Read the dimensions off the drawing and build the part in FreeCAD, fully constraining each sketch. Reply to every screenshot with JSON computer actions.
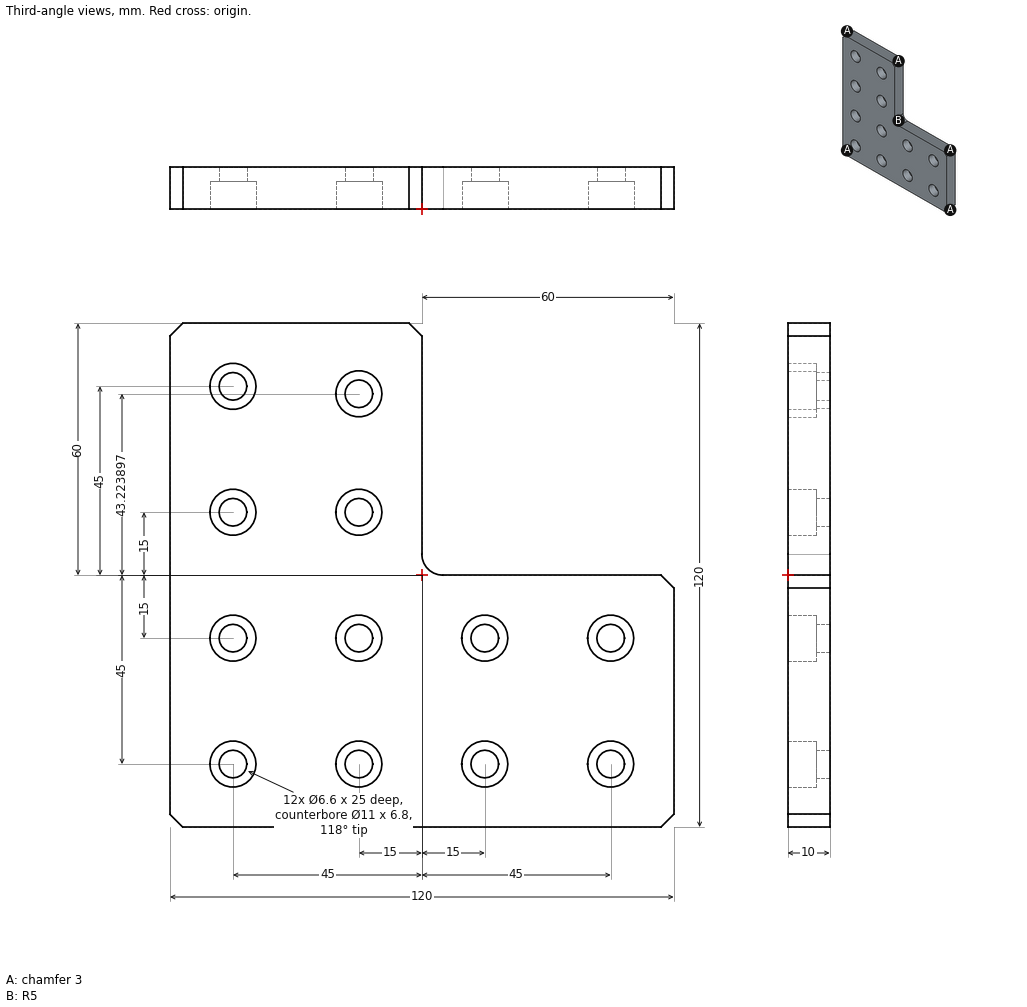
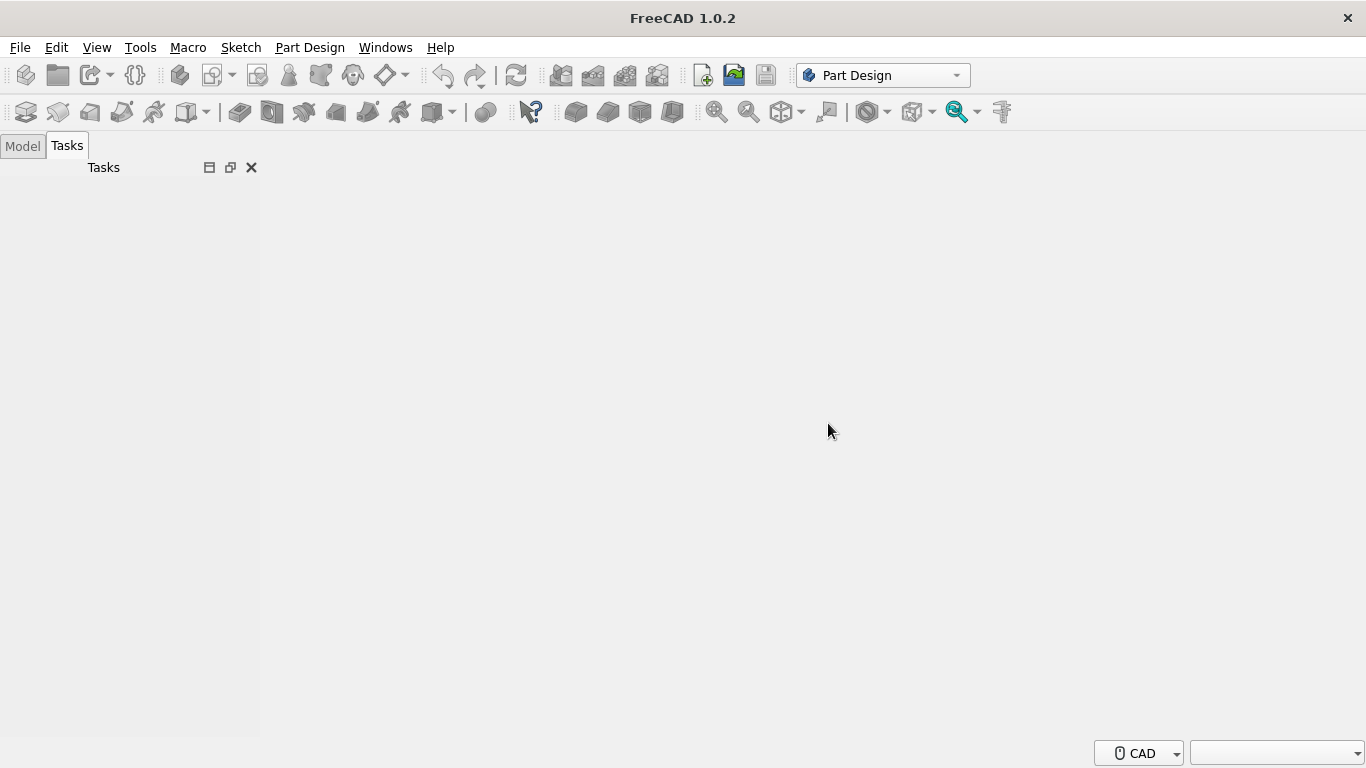
{"action": "left_click", "coordinate": [702, 76]}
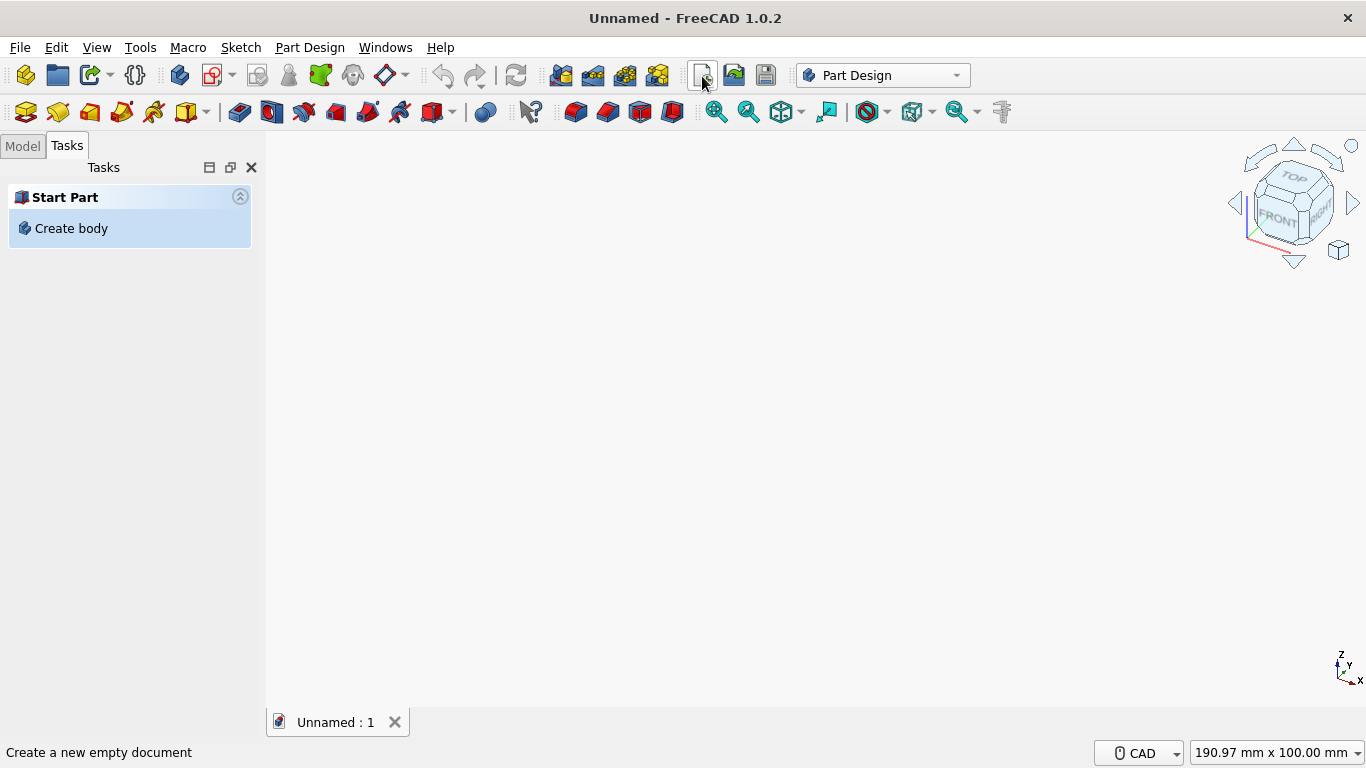
{"action": "left_click", "coordinate": [212, 76]}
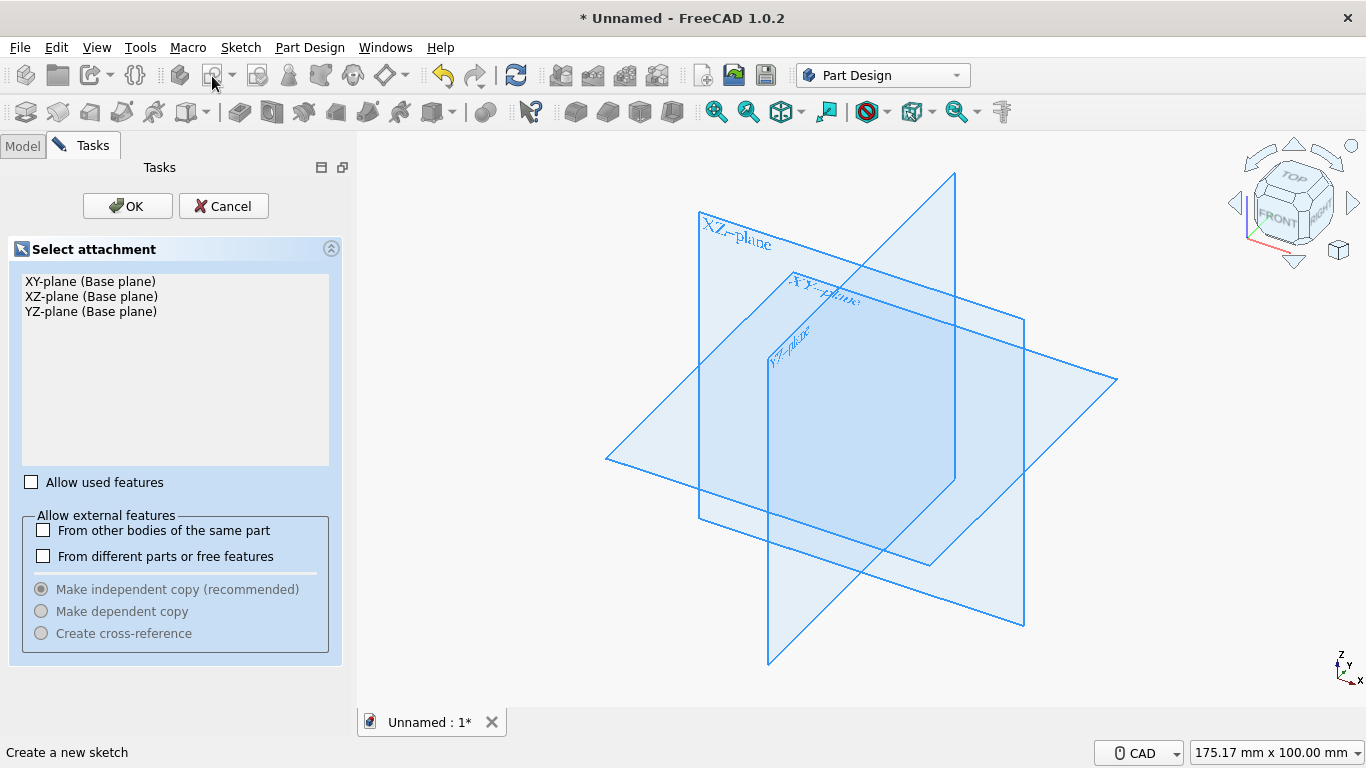
{"action": "left_click", "coordinate": [82, 296]}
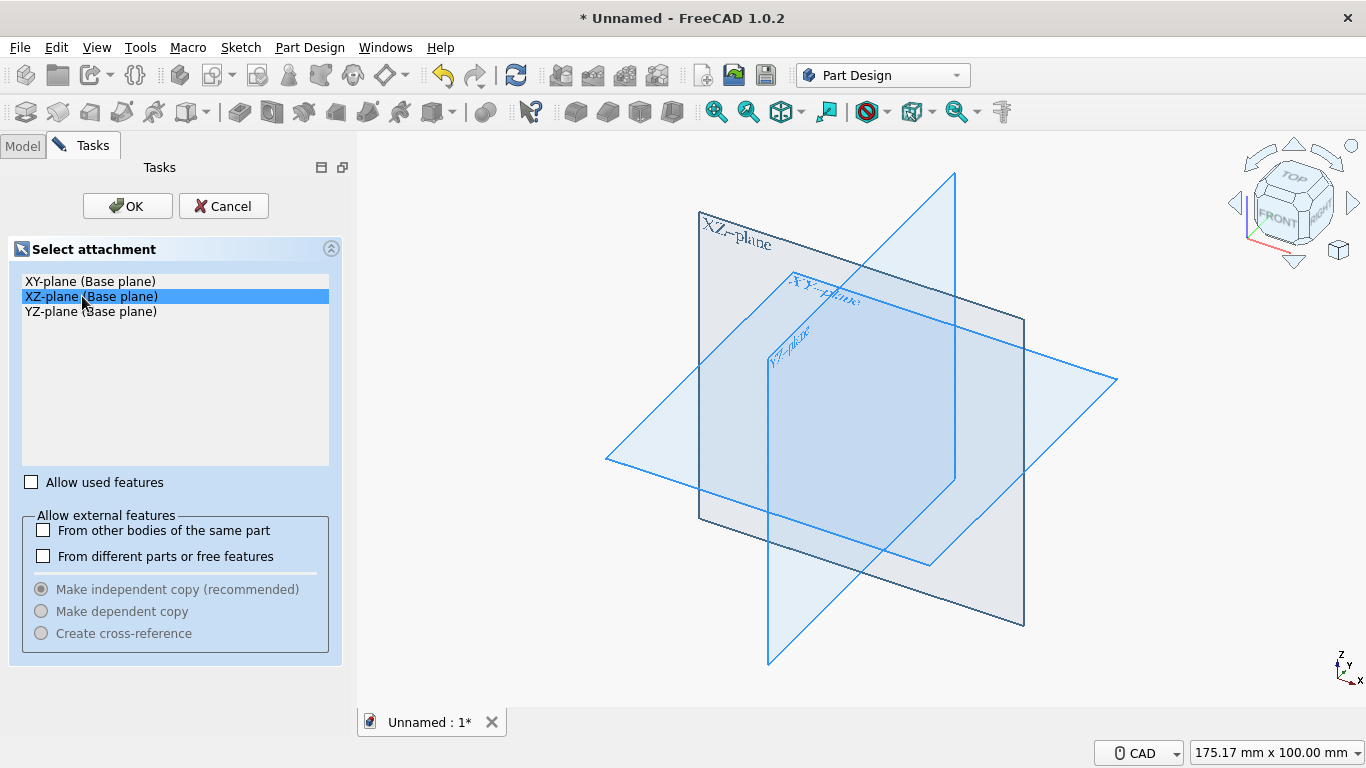
{"action": "left_click", "coordinate": [128, 206]}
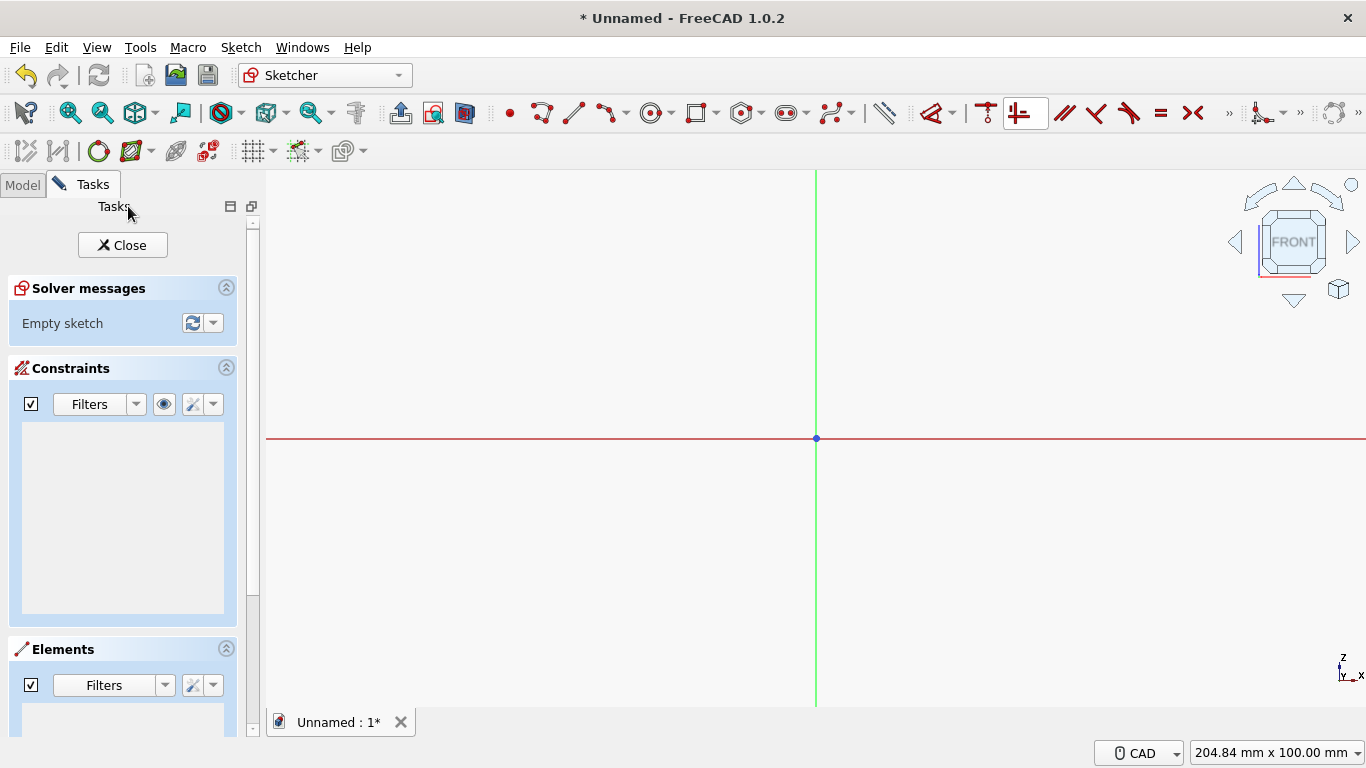
{"action": "scroll", "coordinate": [664, 438], "scroll_direction": "down", "scroll_amount": 3}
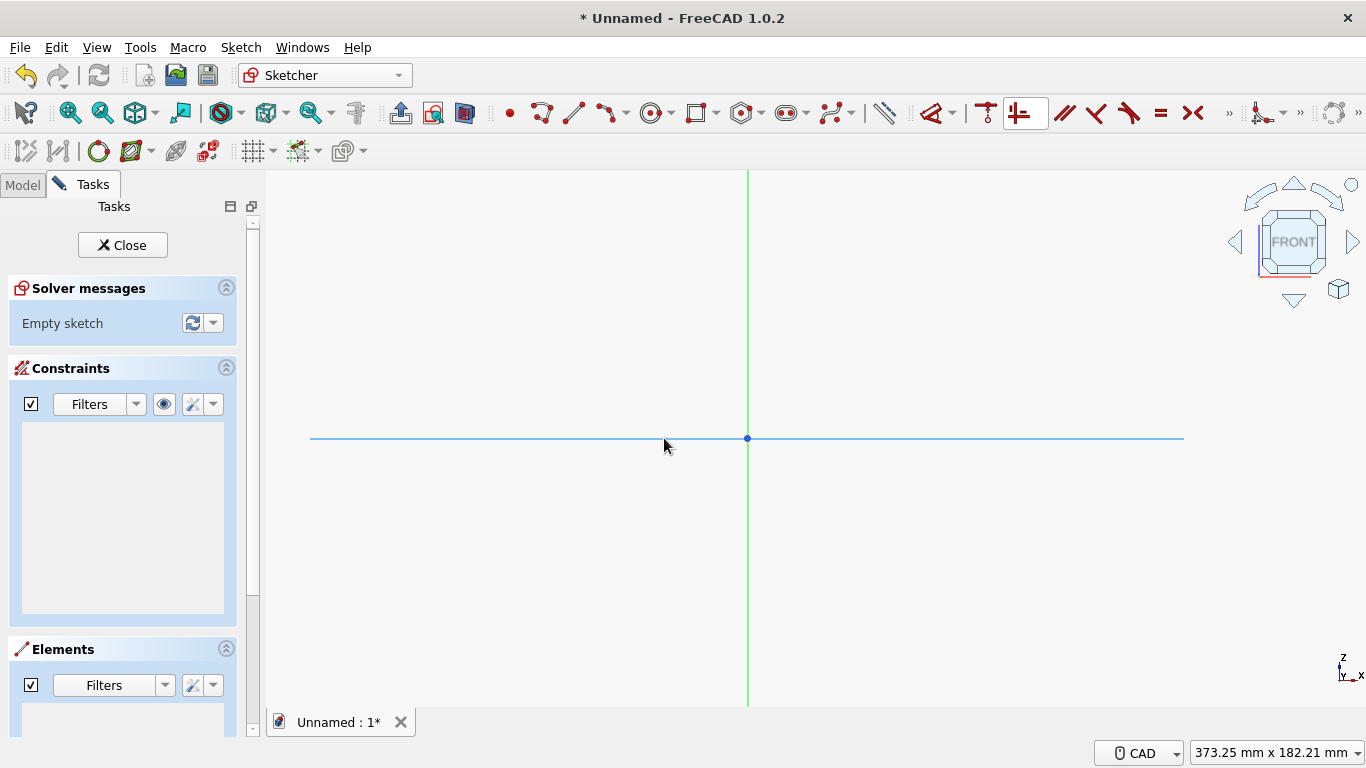
{"action": "key", "text": "g v"}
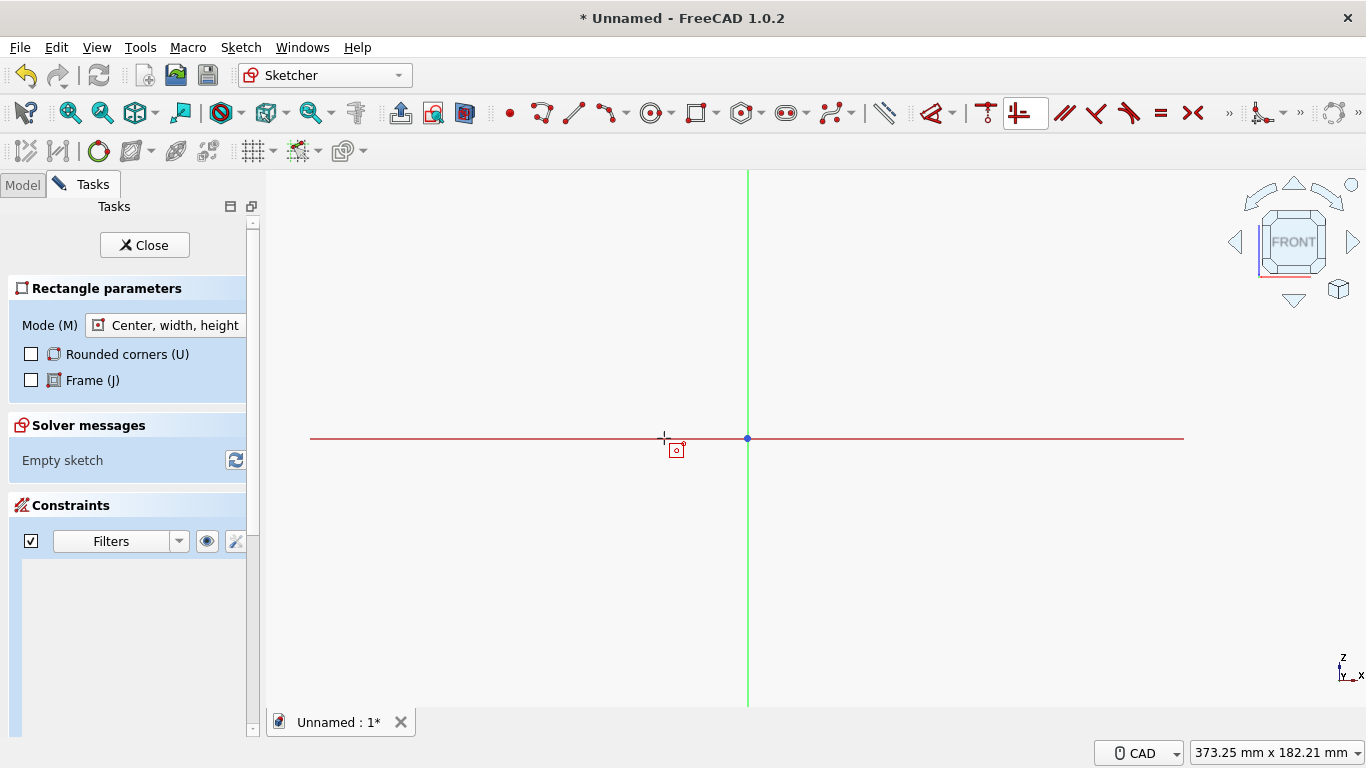
{"action": "left_click", "coordinate": [748, 438]}
{"action": "left_click", "coordinate": [924, 262]}
{"action": "key", "text": "Escape"}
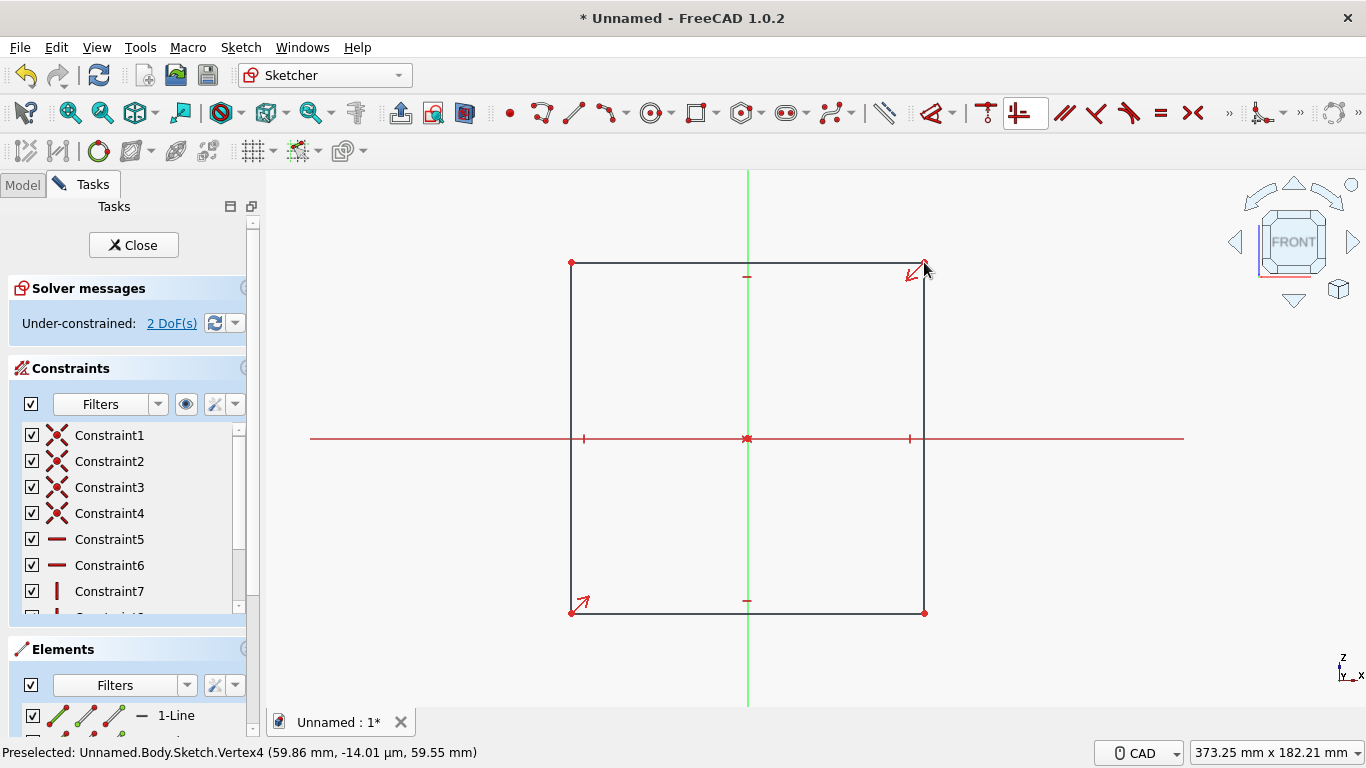
{"action": "left_click", "coordinate": [932, 114]}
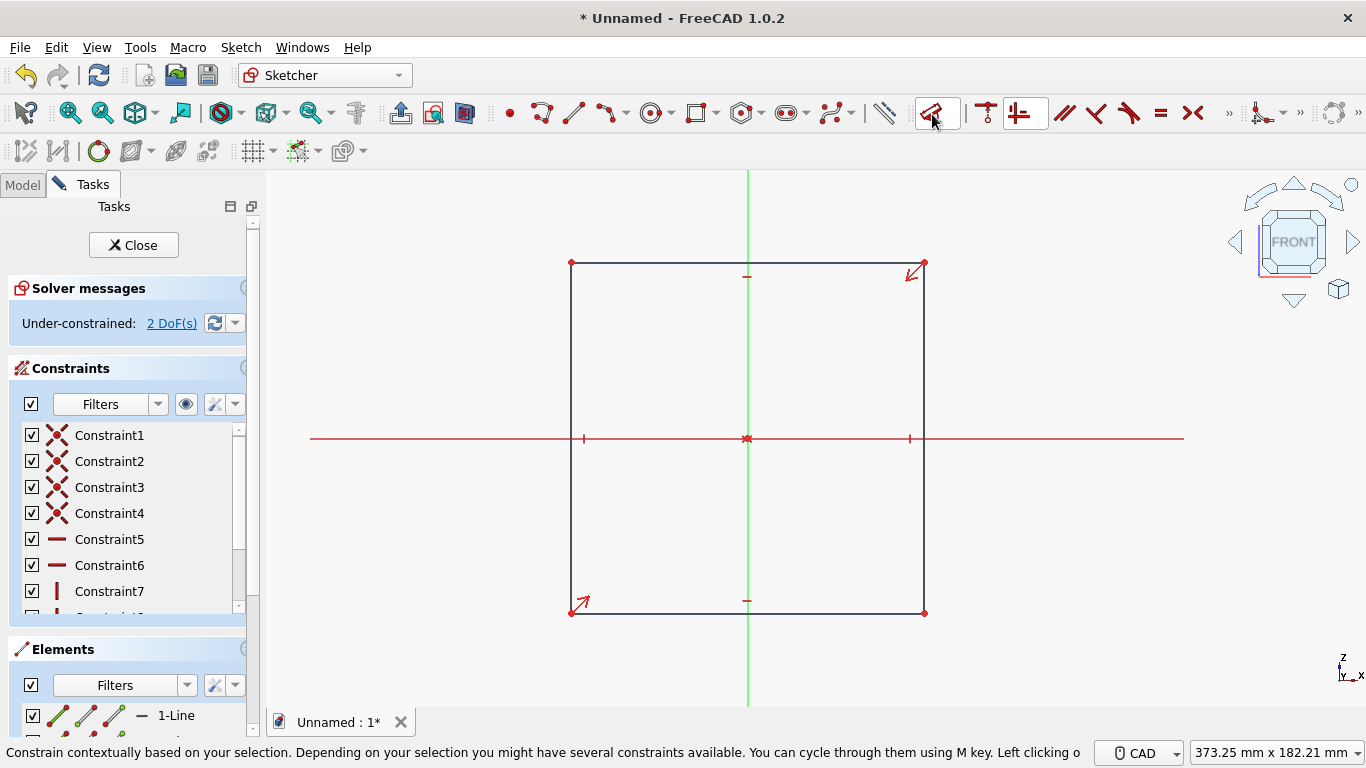
{"action": "left_click", "coordinate": [677, 614]}
{"action": "left_click", "coordinate": [666, 648]}